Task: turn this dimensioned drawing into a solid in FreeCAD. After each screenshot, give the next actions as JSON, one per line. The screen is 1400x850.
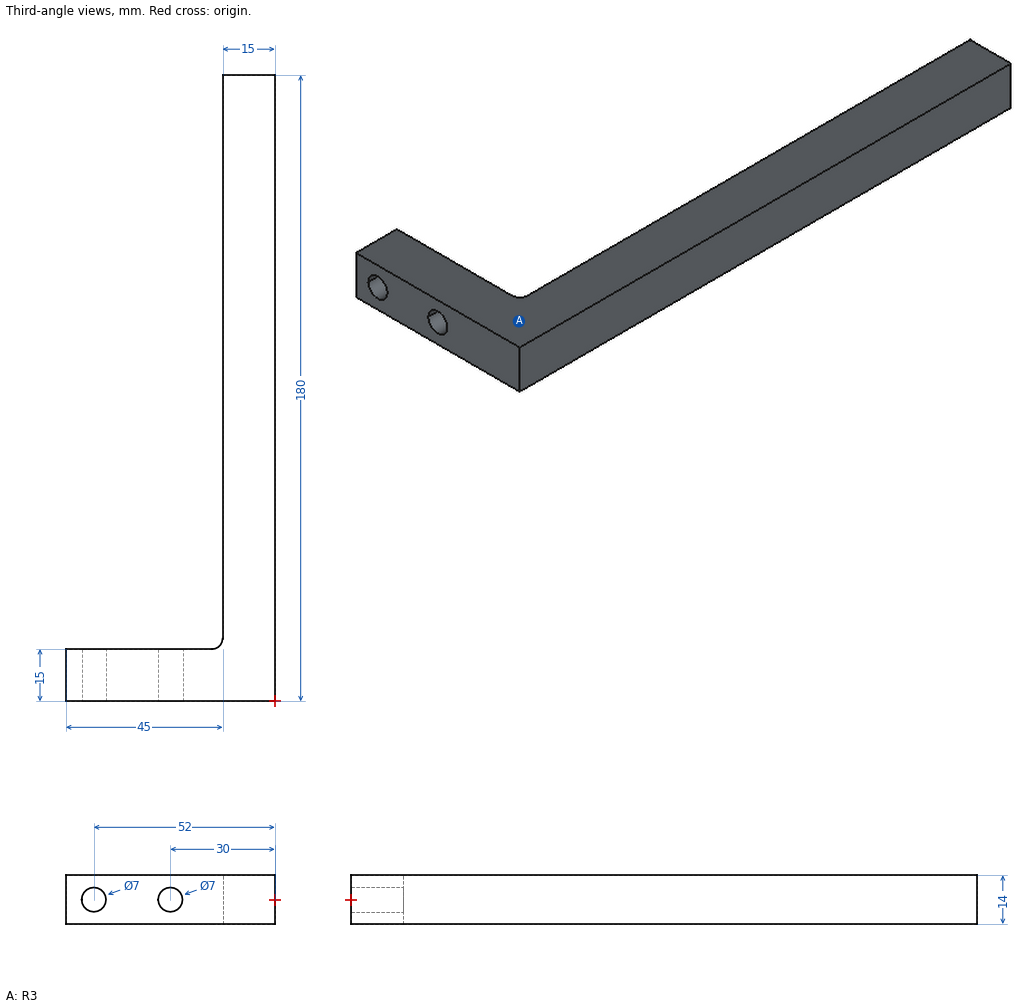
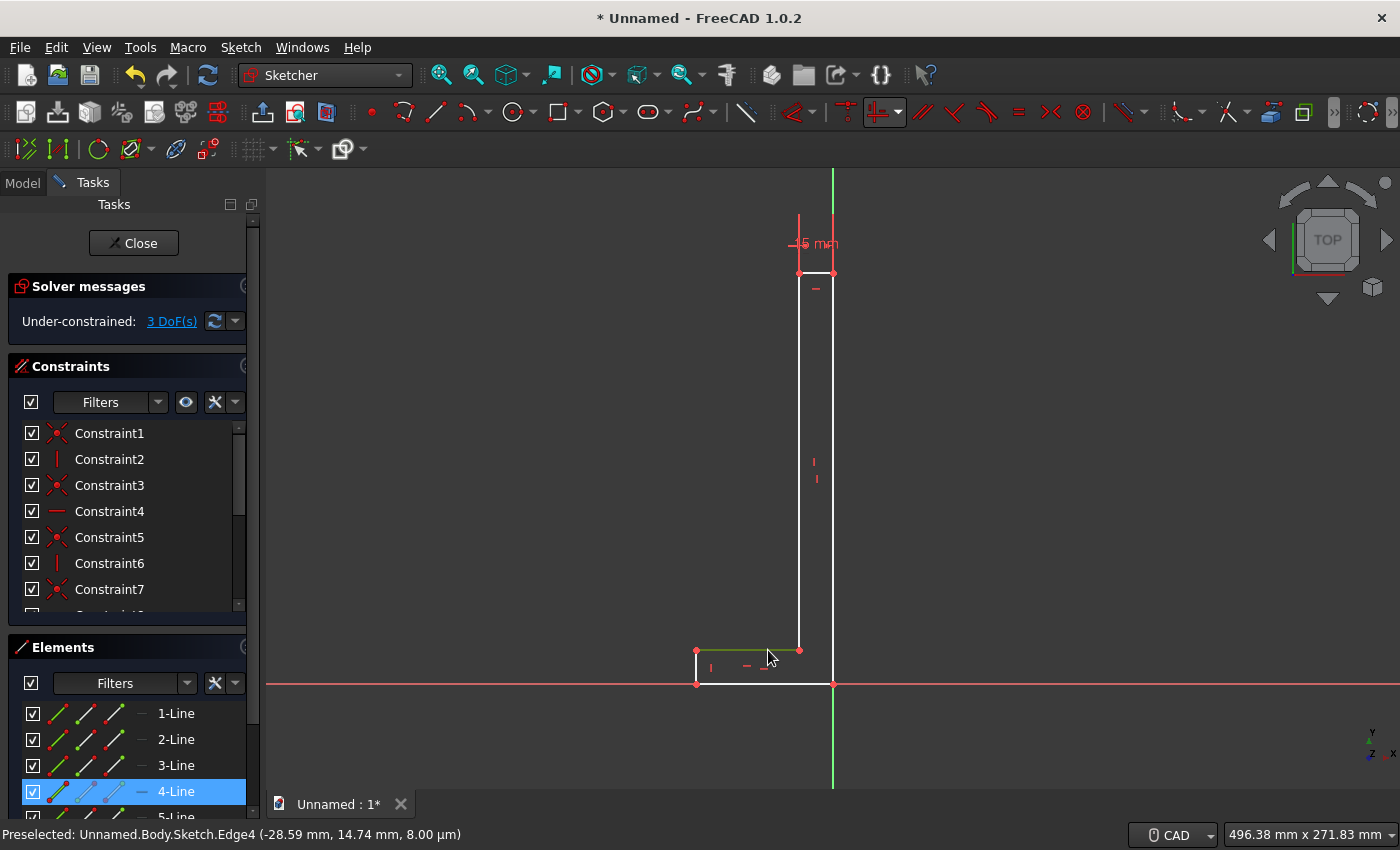
{"action": "key", "text": "l"}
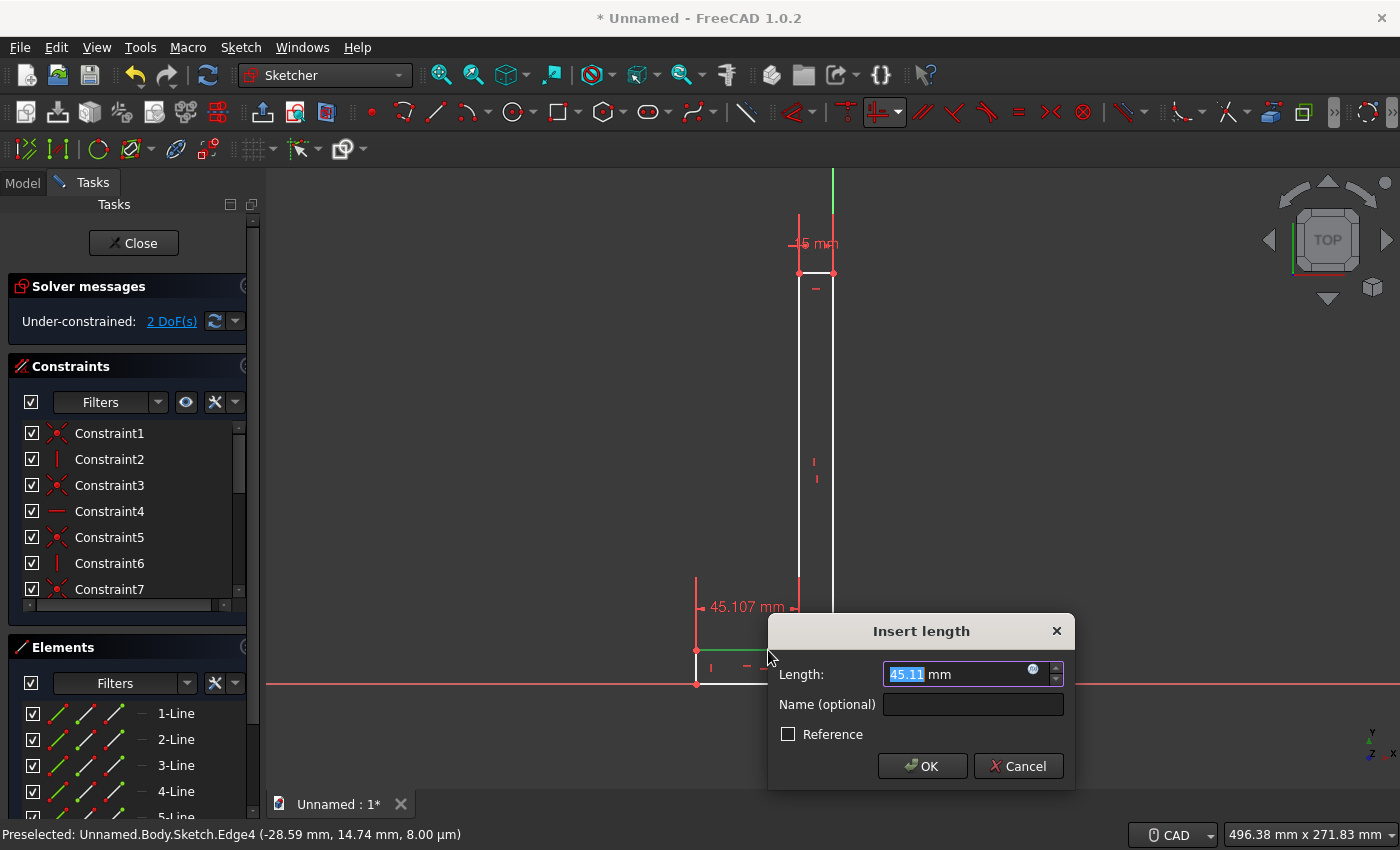
{"action": "type", "text": "45"}
{"action": "key", "text": "Return"}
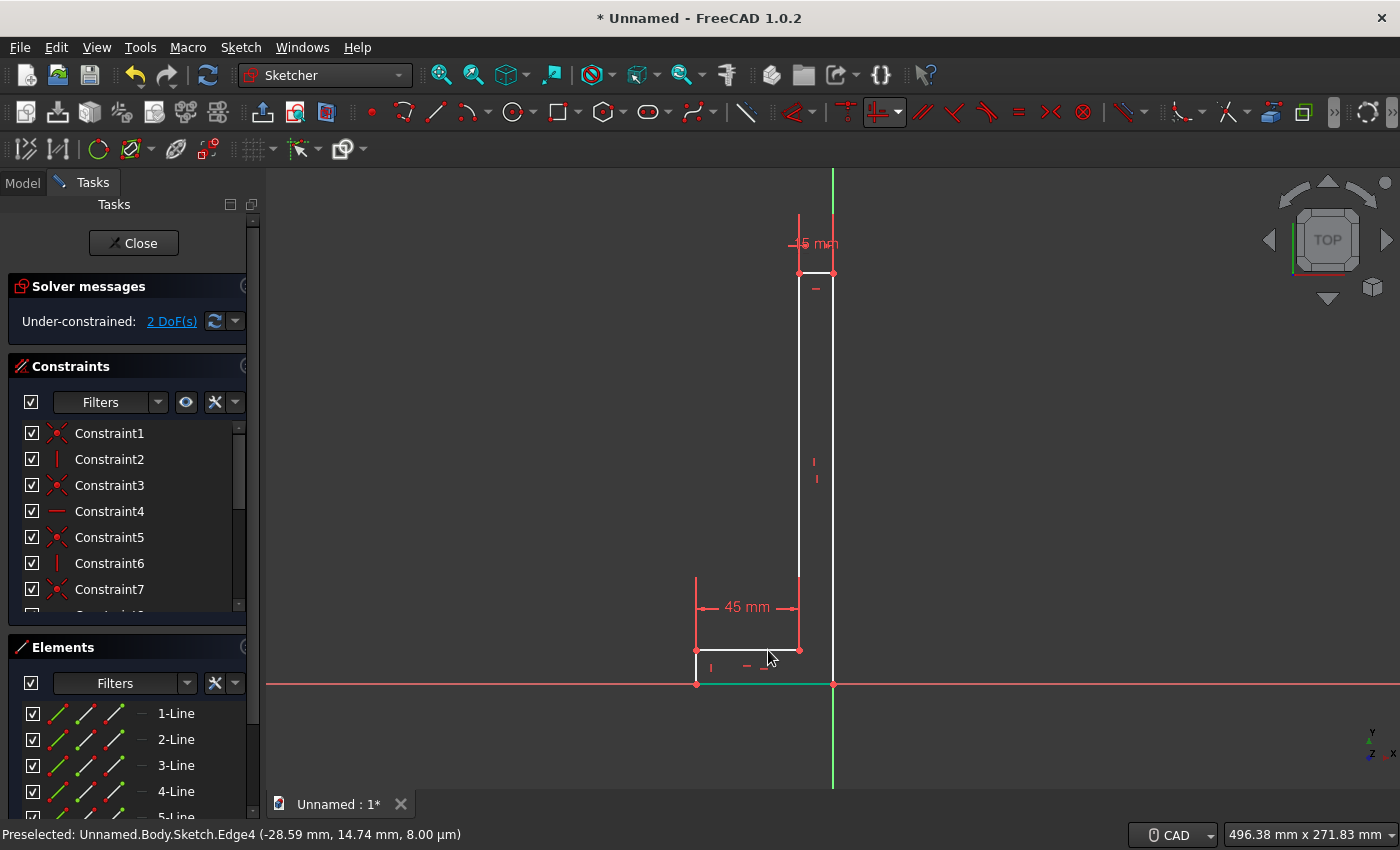
{"action": "scroll", "coordinate": [696, 661], "scroll_direction": "up", "scroll_amount": 2}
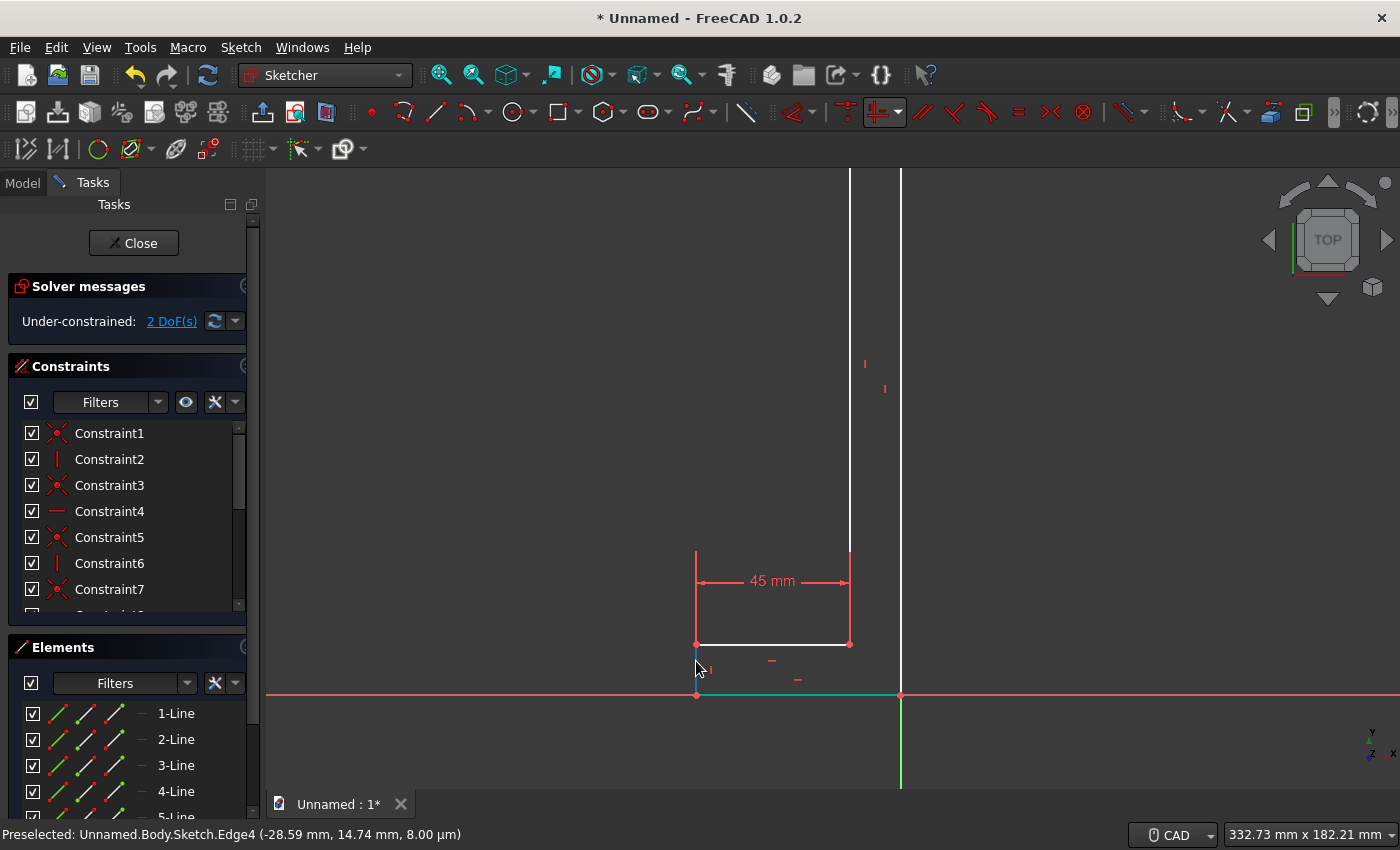
{"action": "left_click", "coordinate": [696, 660]}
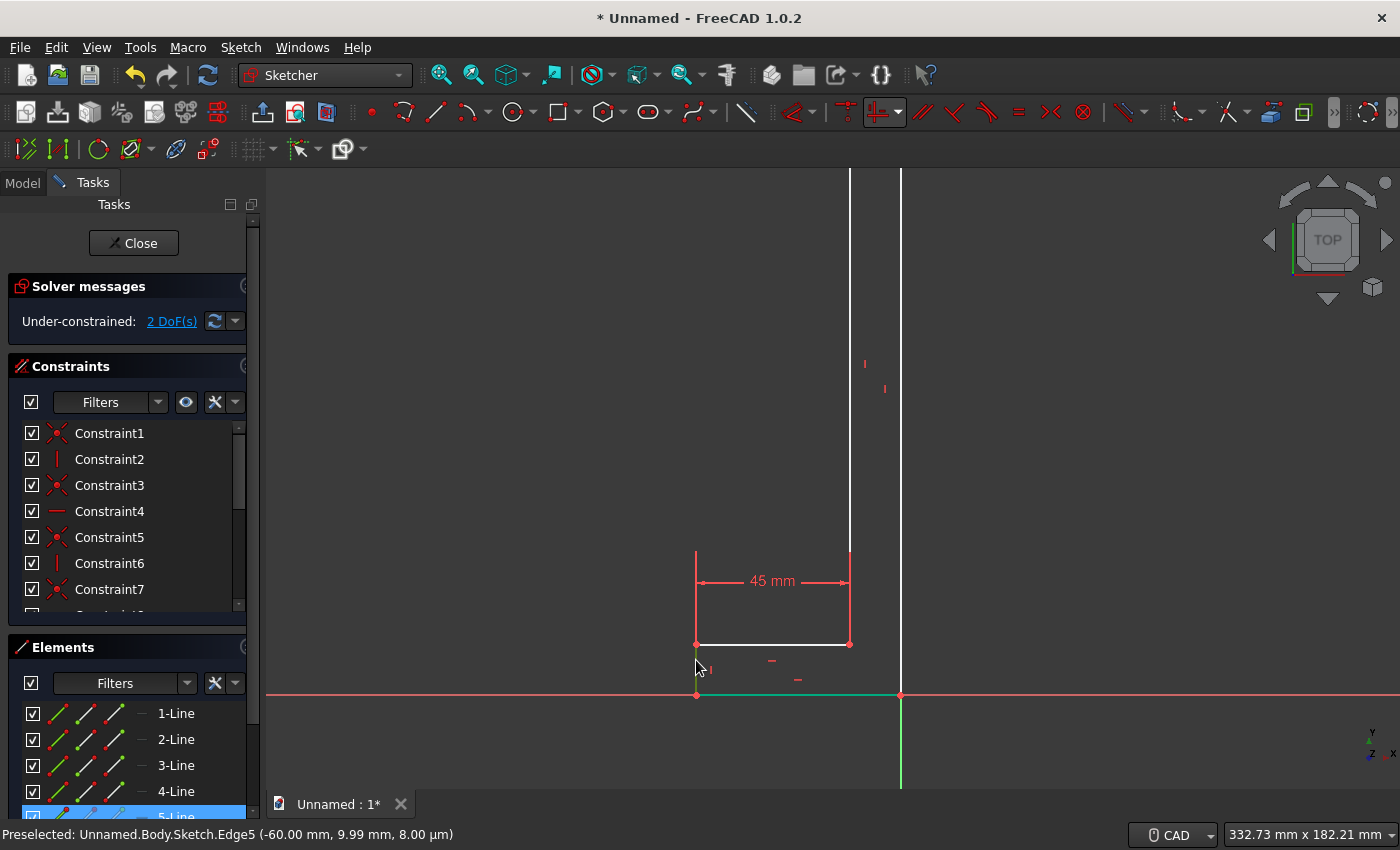
{"action": "key", "text": "i"}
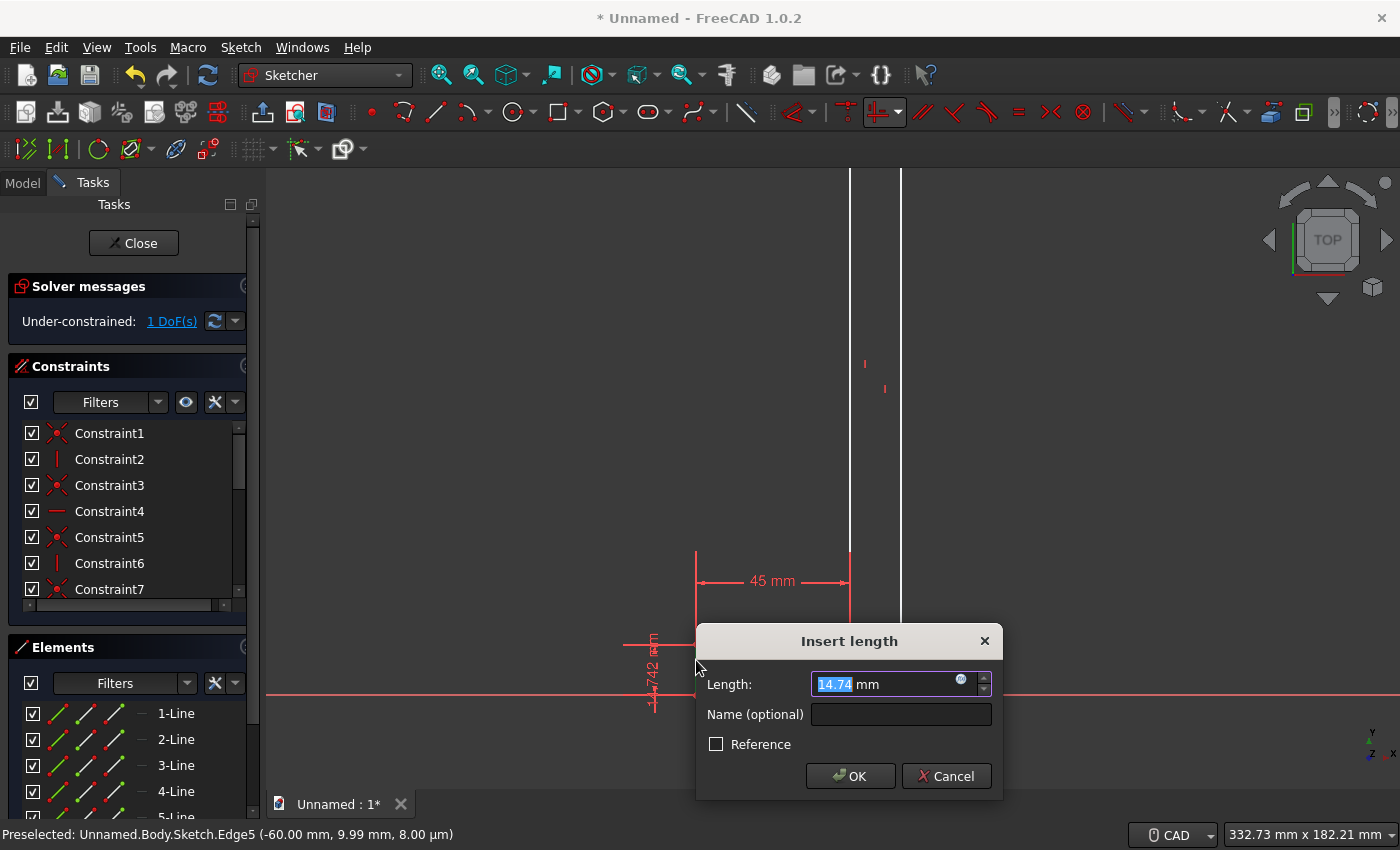
{"action": "type", "text": "15"}
{"action": "key", "text": "Return"}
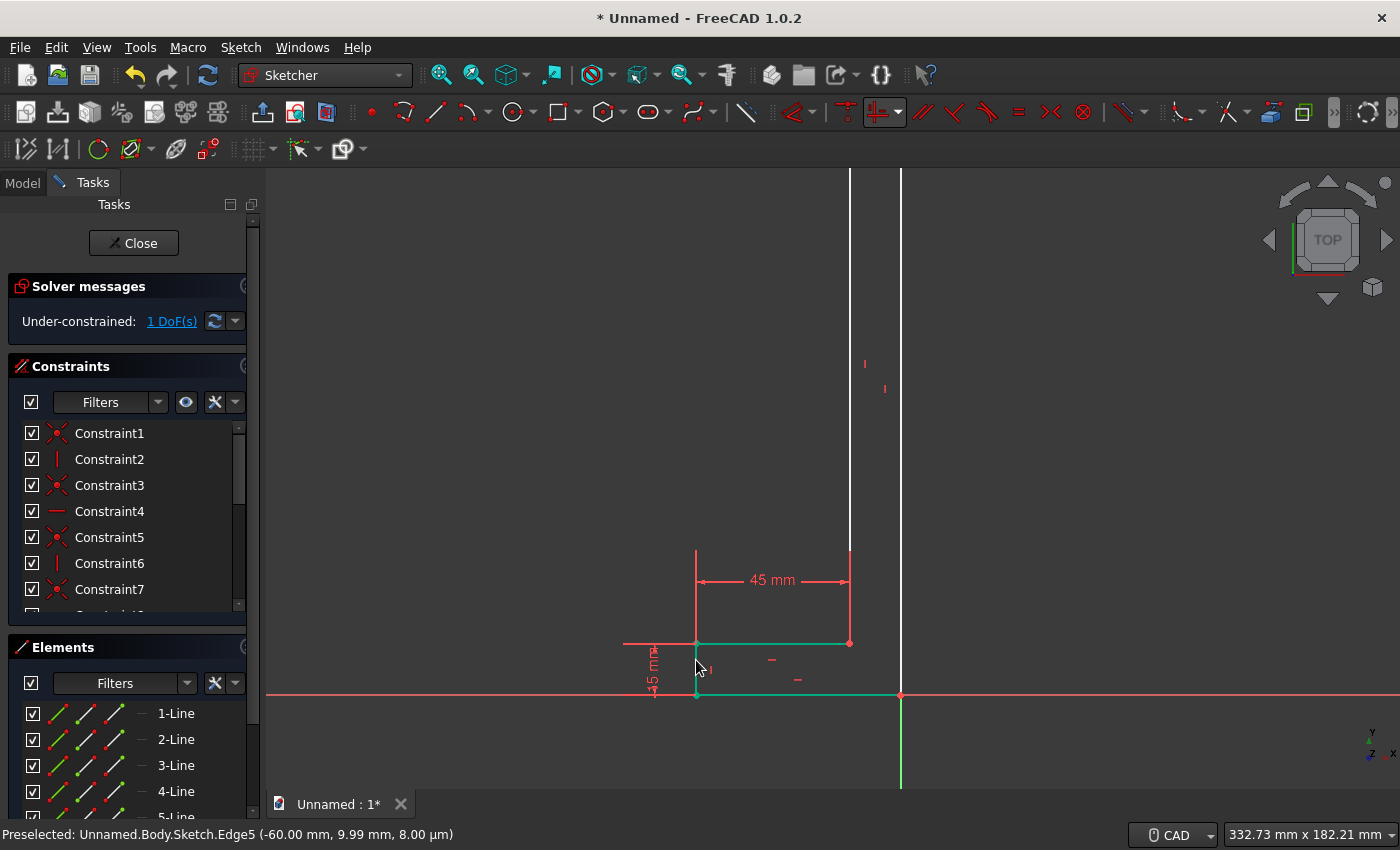
{"action": "left_click", "coordinate": [901, 511]}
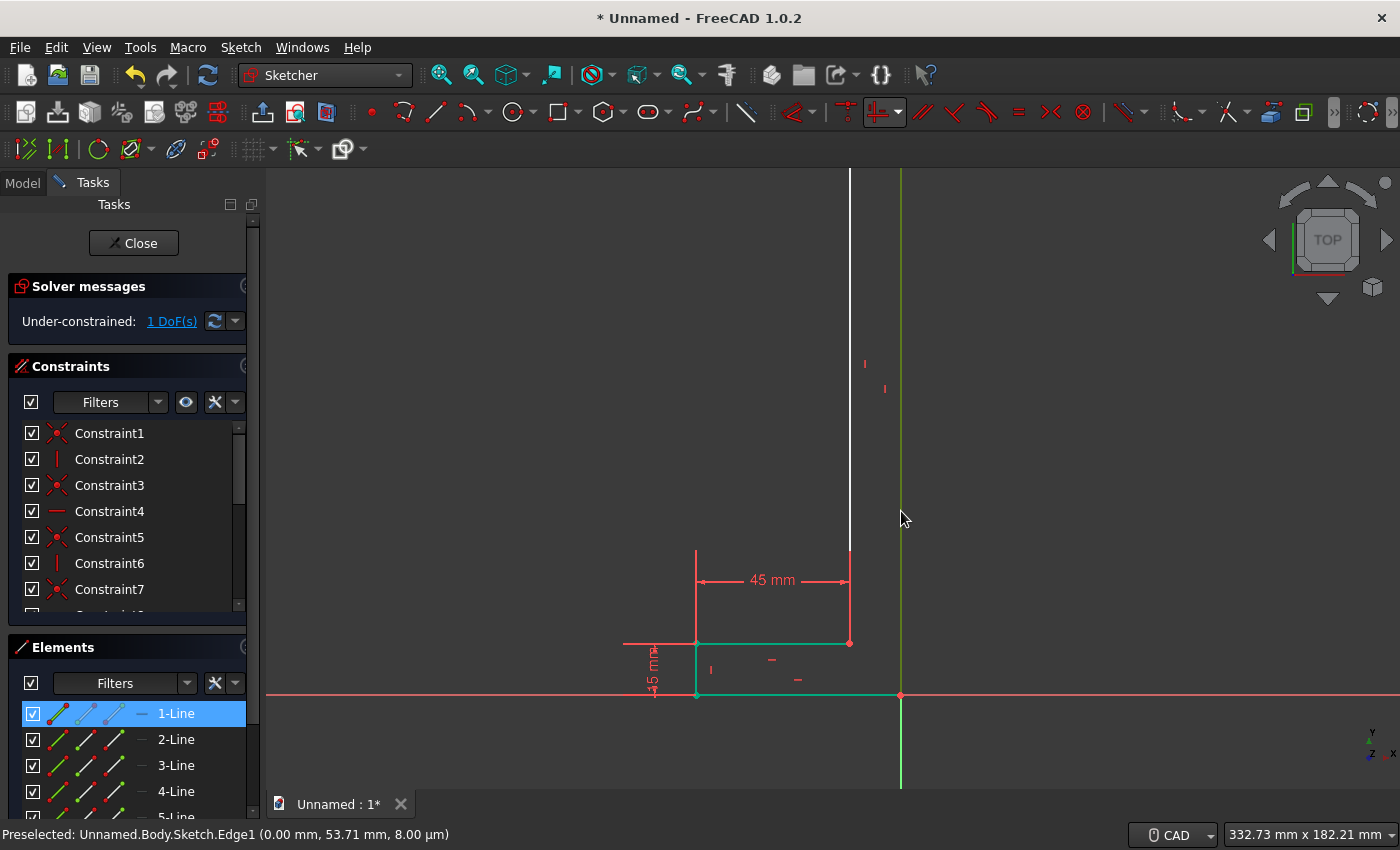
{"action": "key", "text": "i"}